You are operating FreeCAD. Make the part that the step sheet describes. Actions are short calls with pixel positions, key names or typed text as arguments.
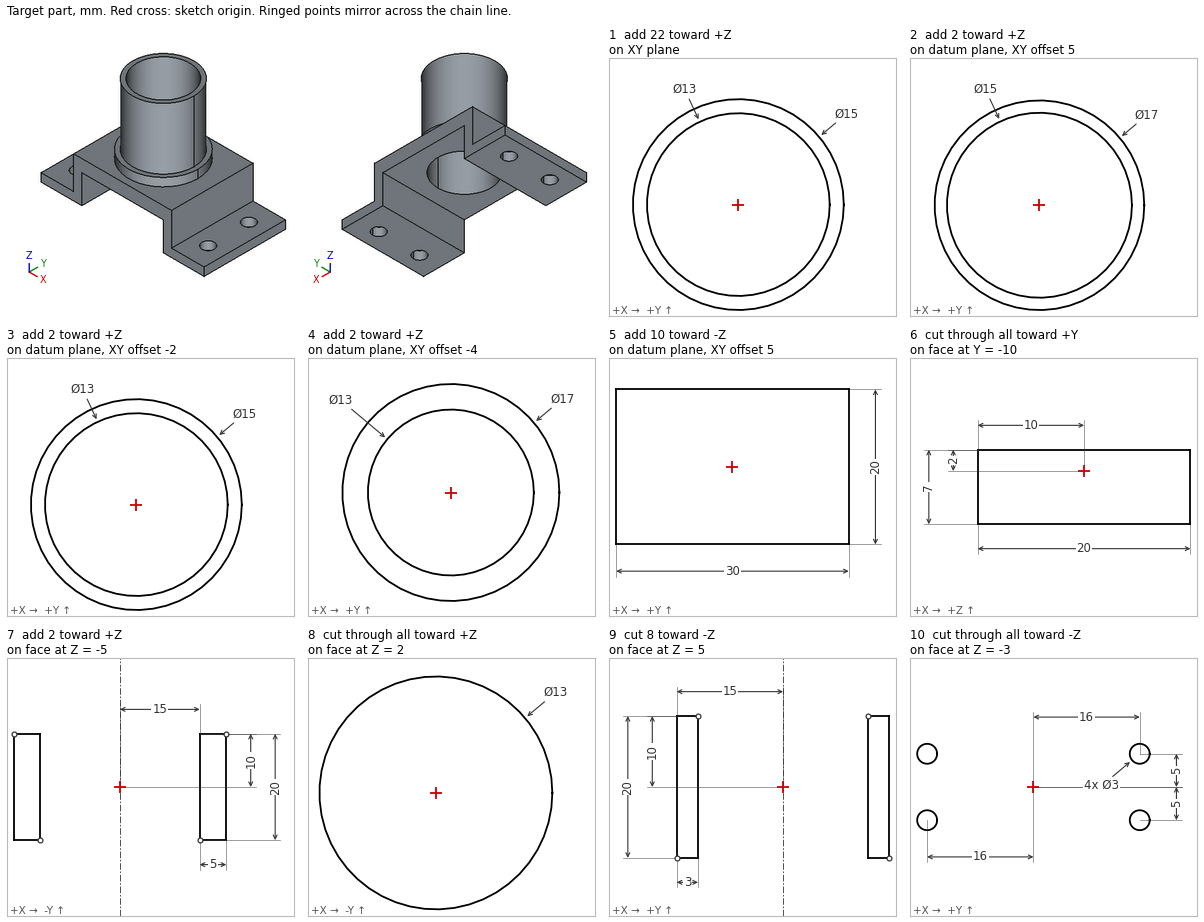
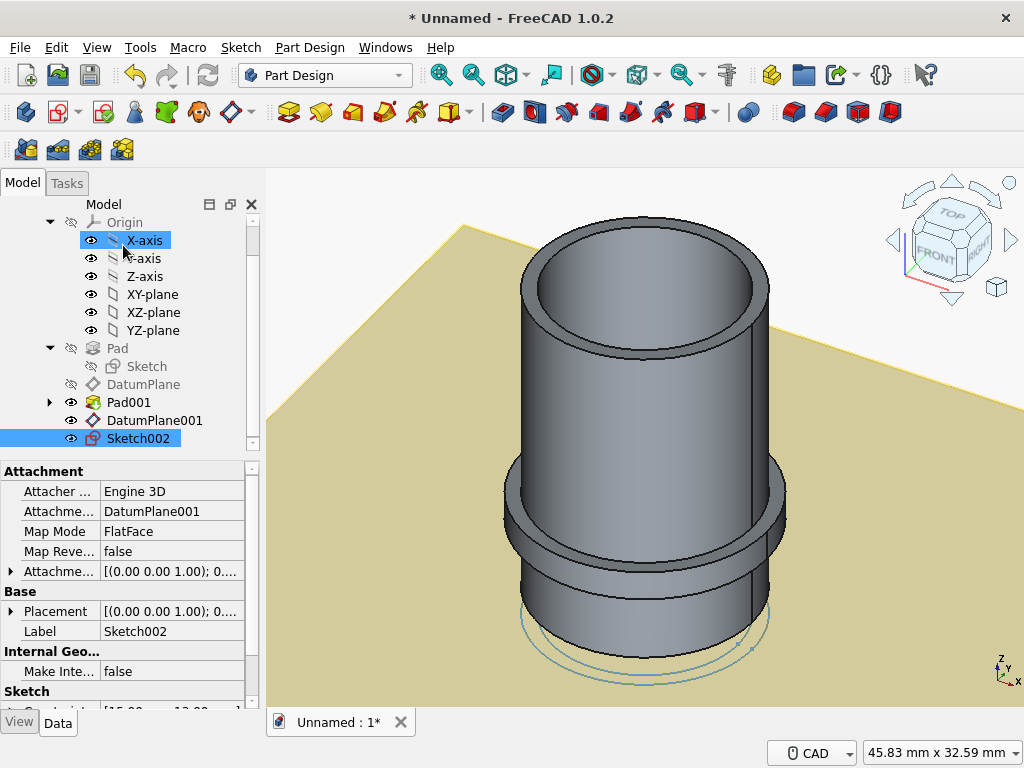
click(290, 112)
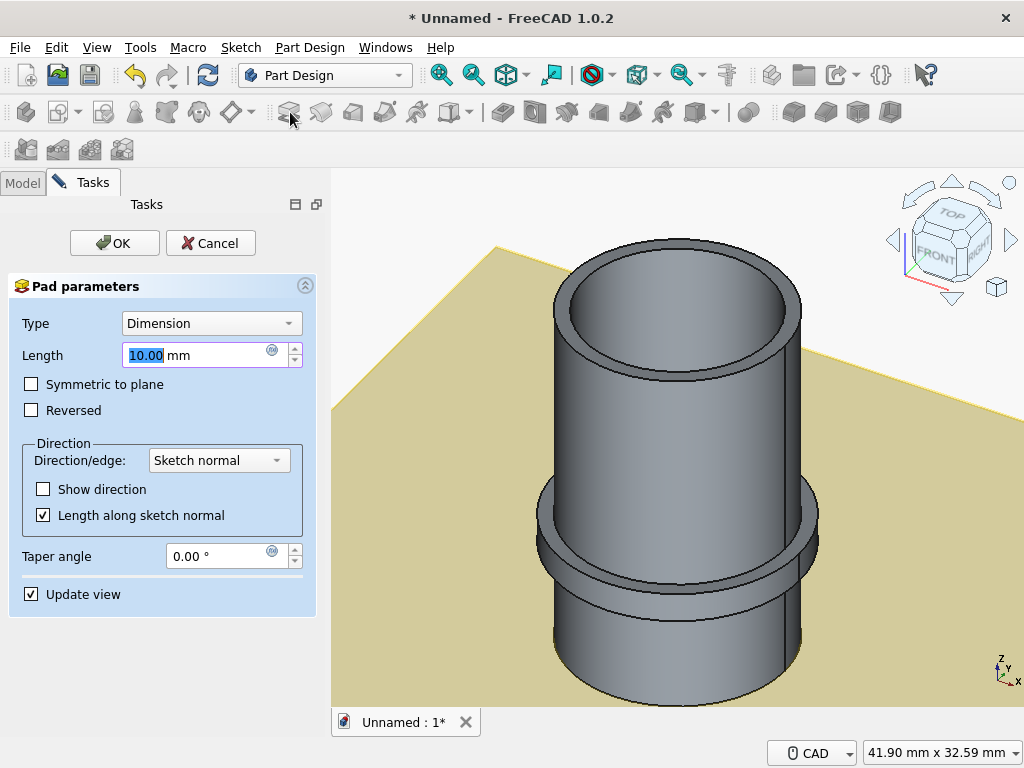
text(2)
key(Tab)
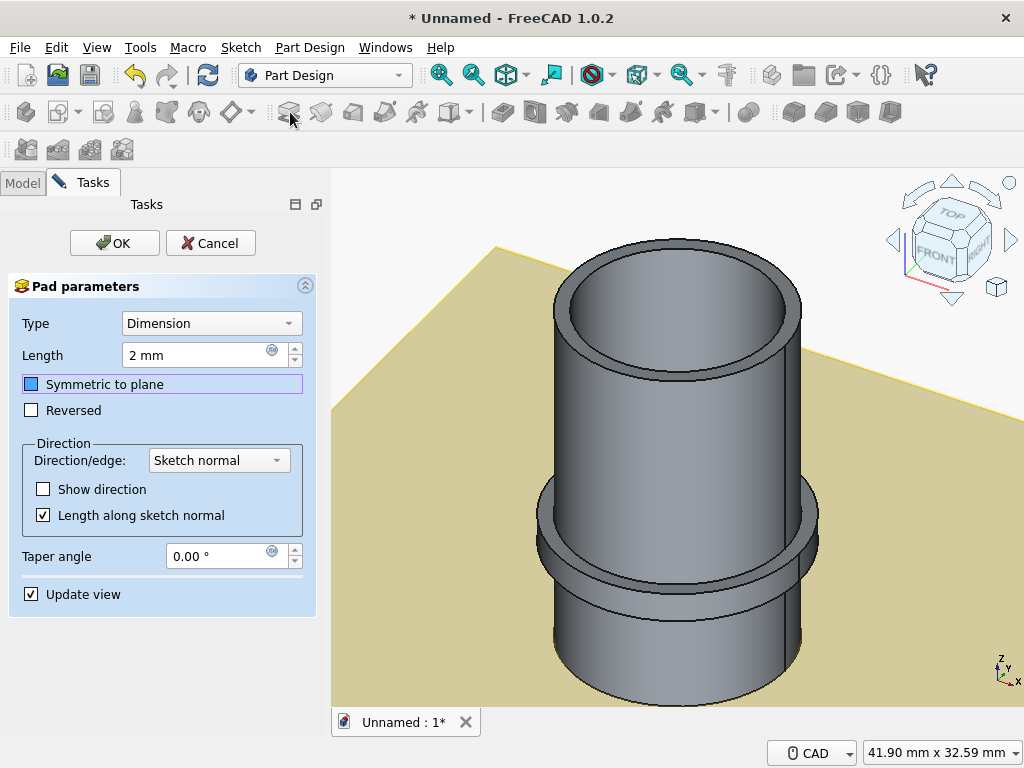
click(115, 243)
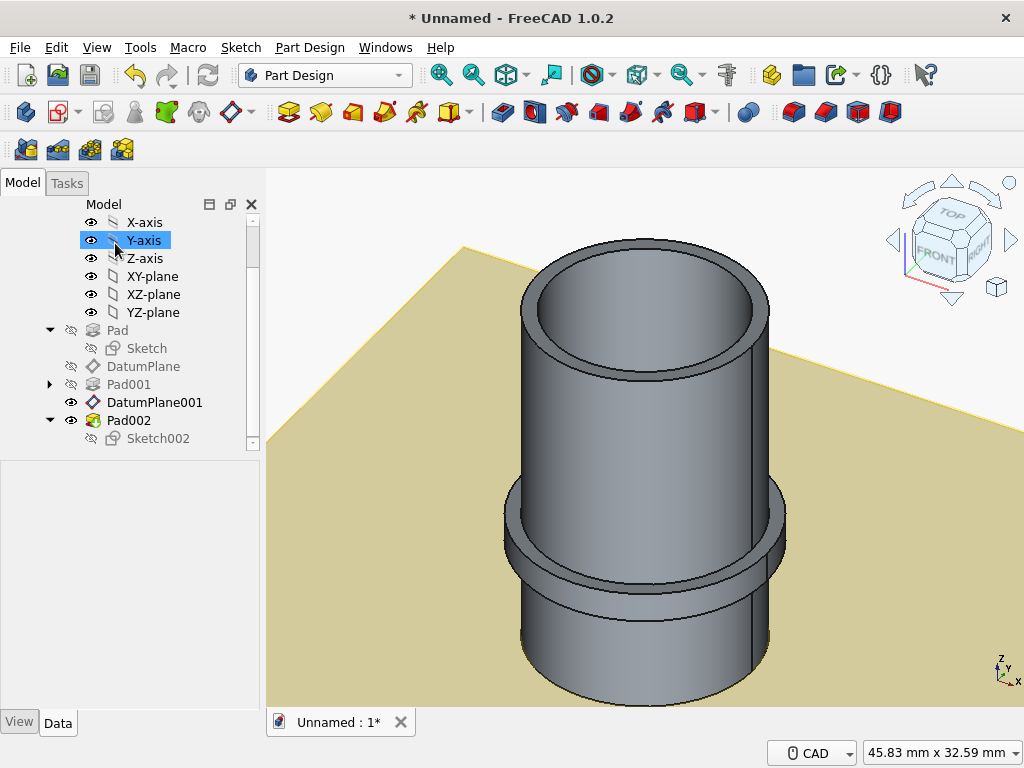
click(116, 402)
key(space)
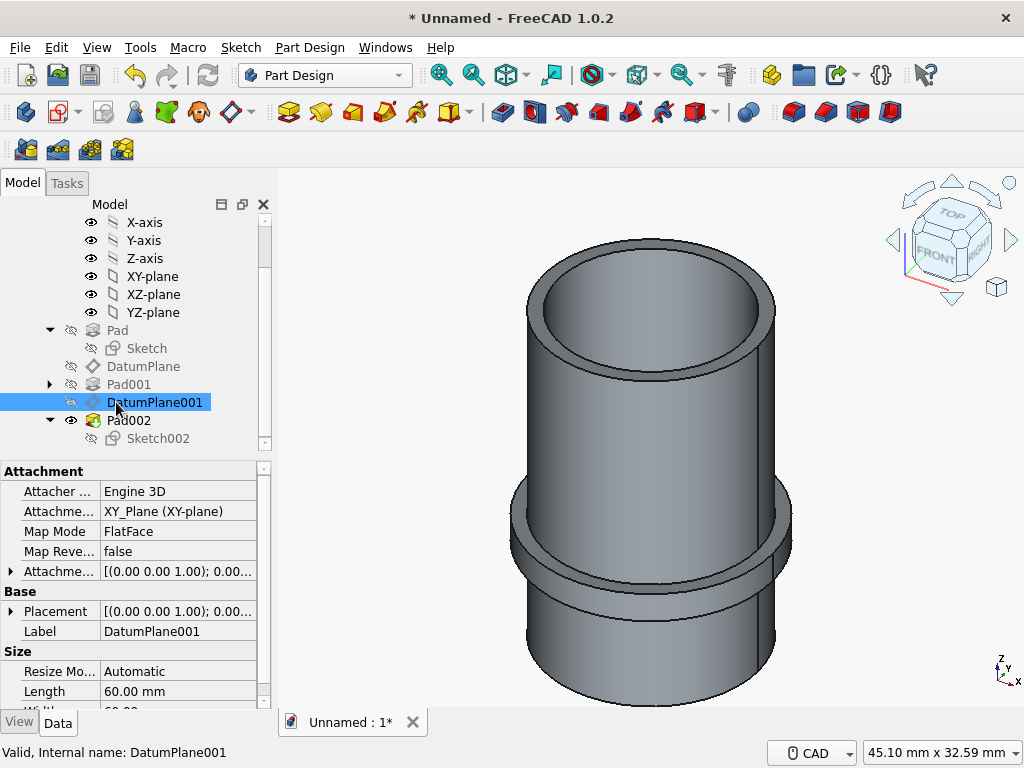
click(442, 76)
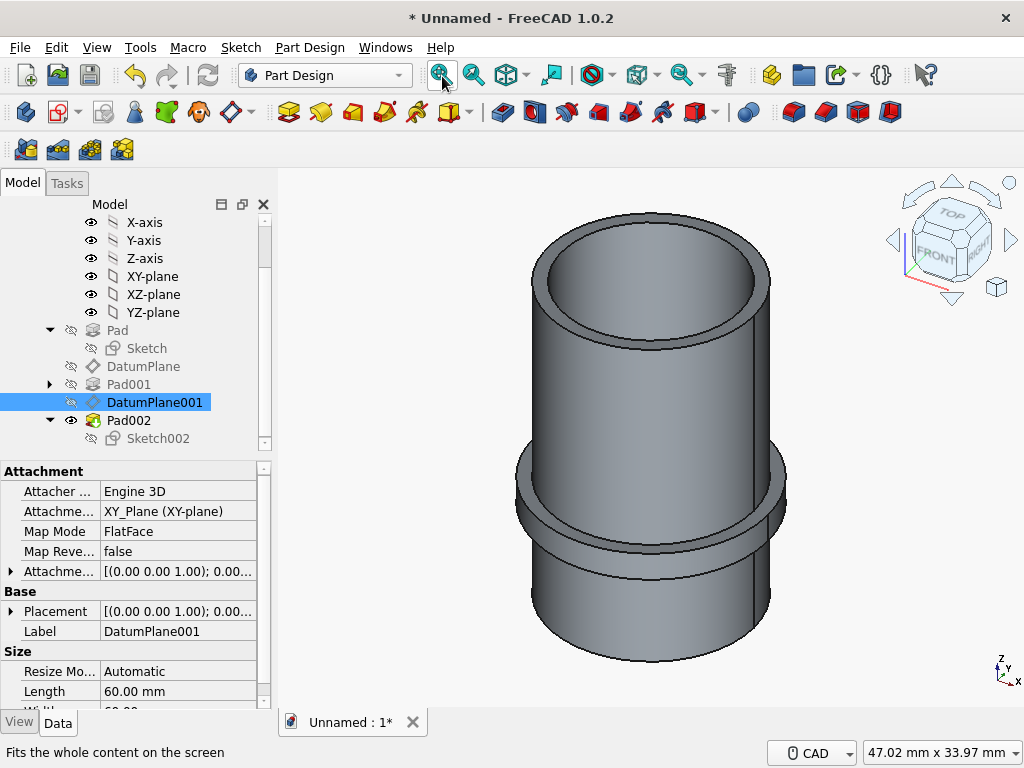
scroll(160, 326, down, 3)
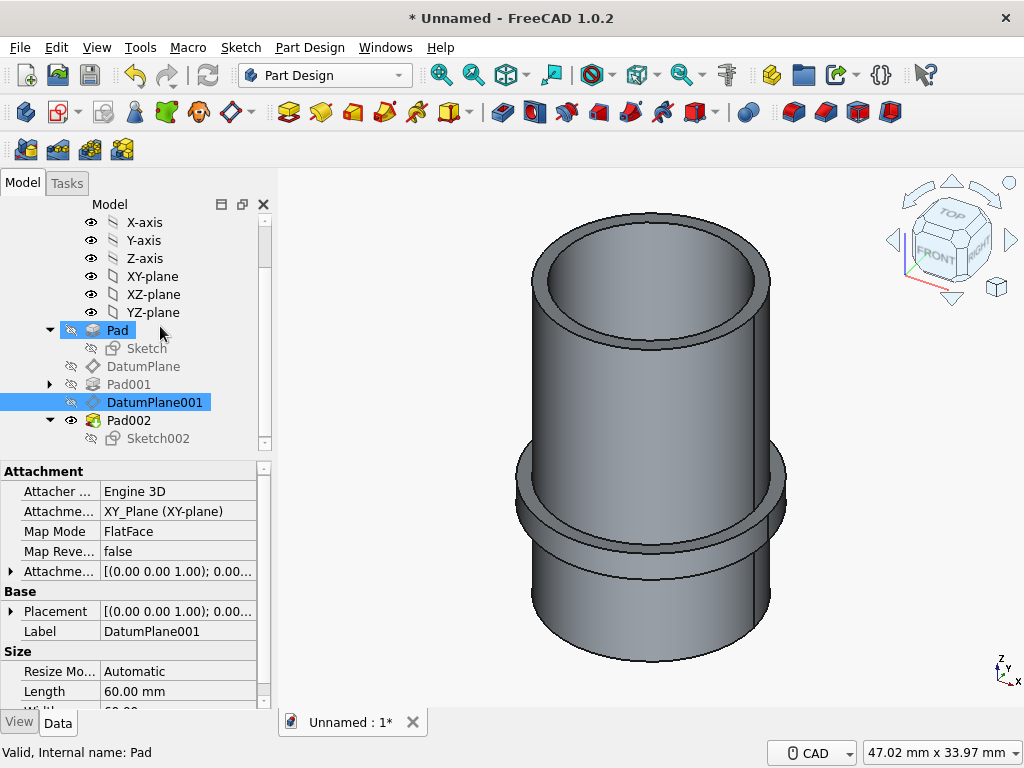
scroll(160, 326, up, 15)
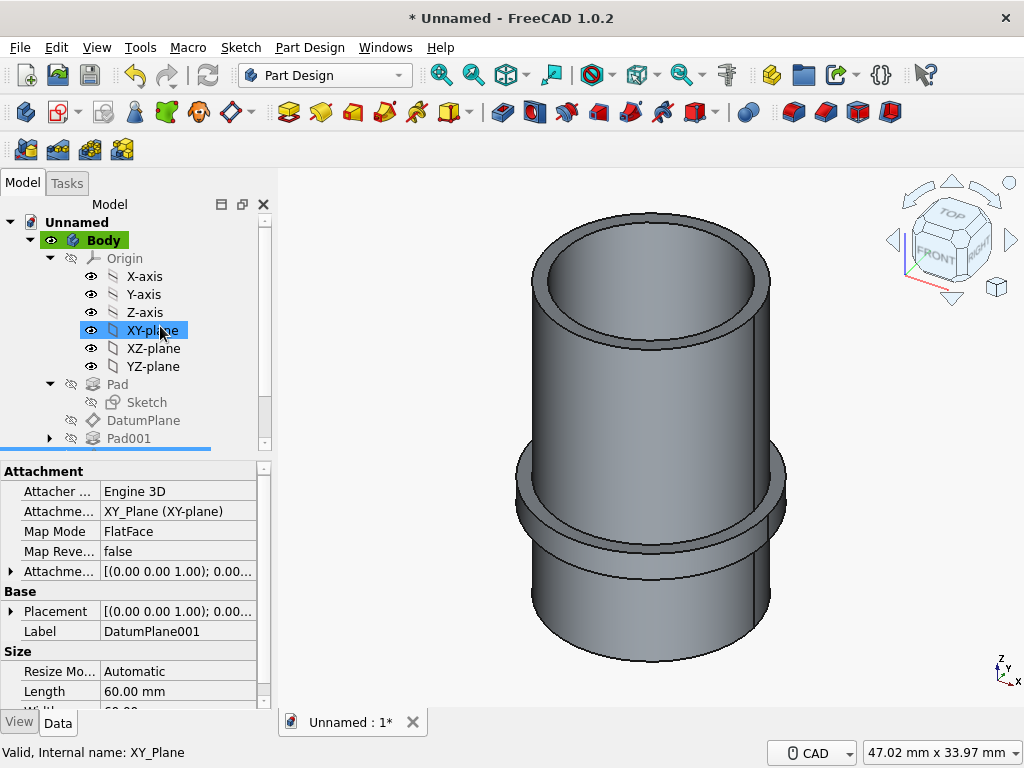
click(136, 330)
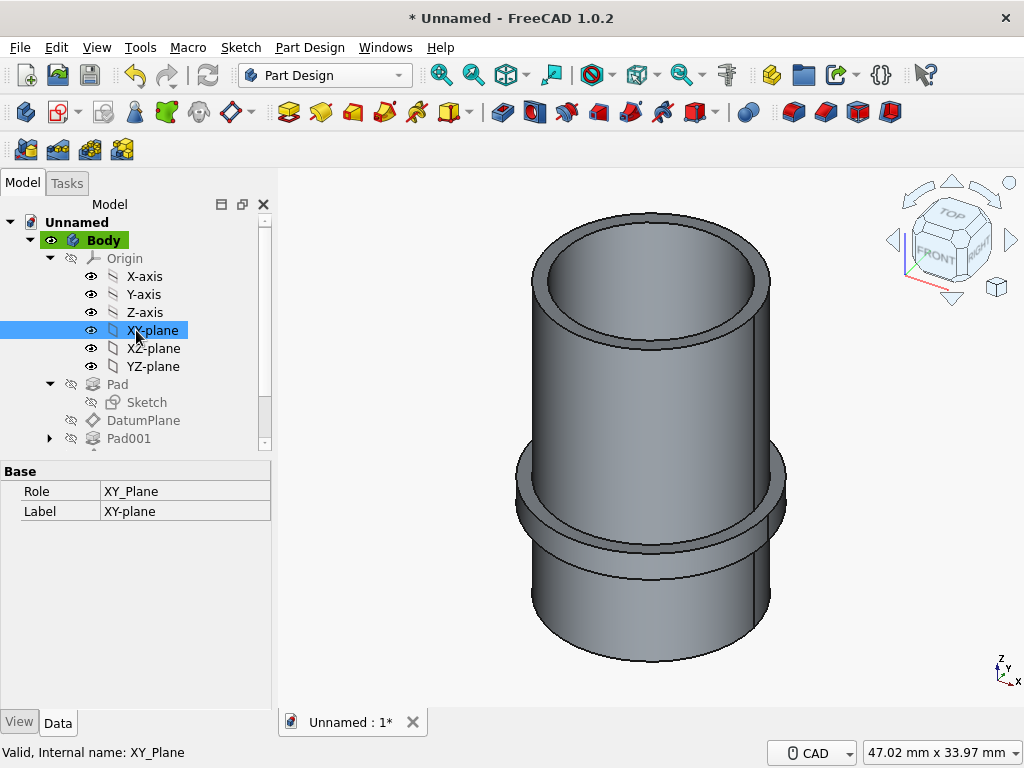
click(232, 112)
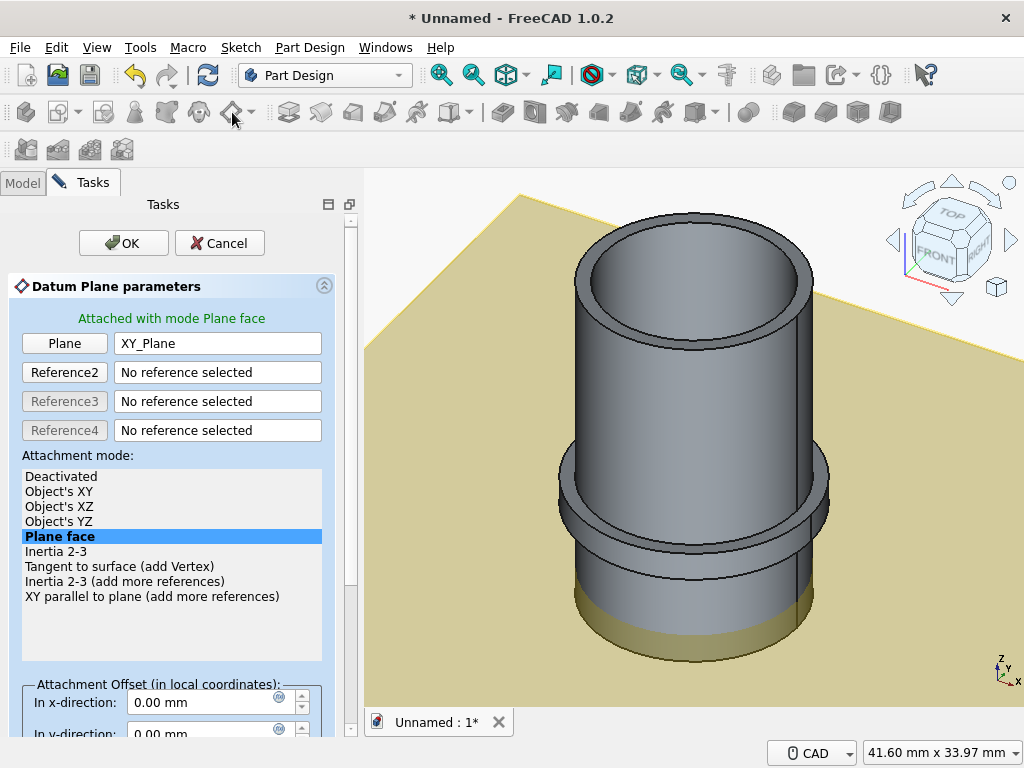
scroll(351, 475, down, 2)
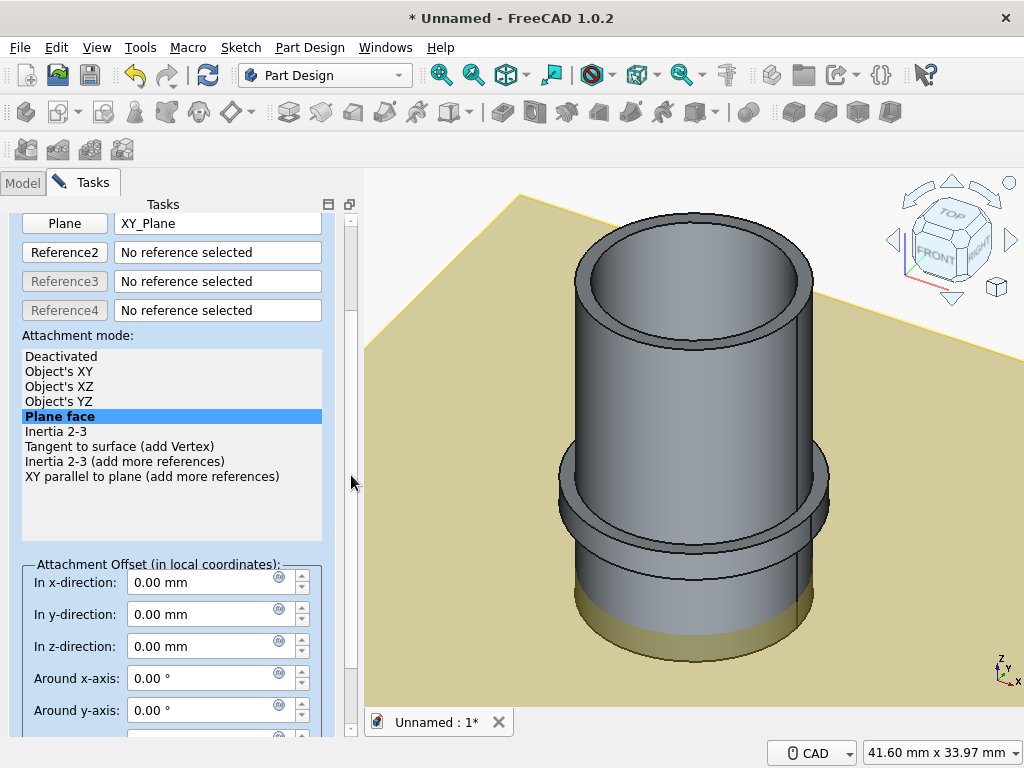
triple_click(210, 646)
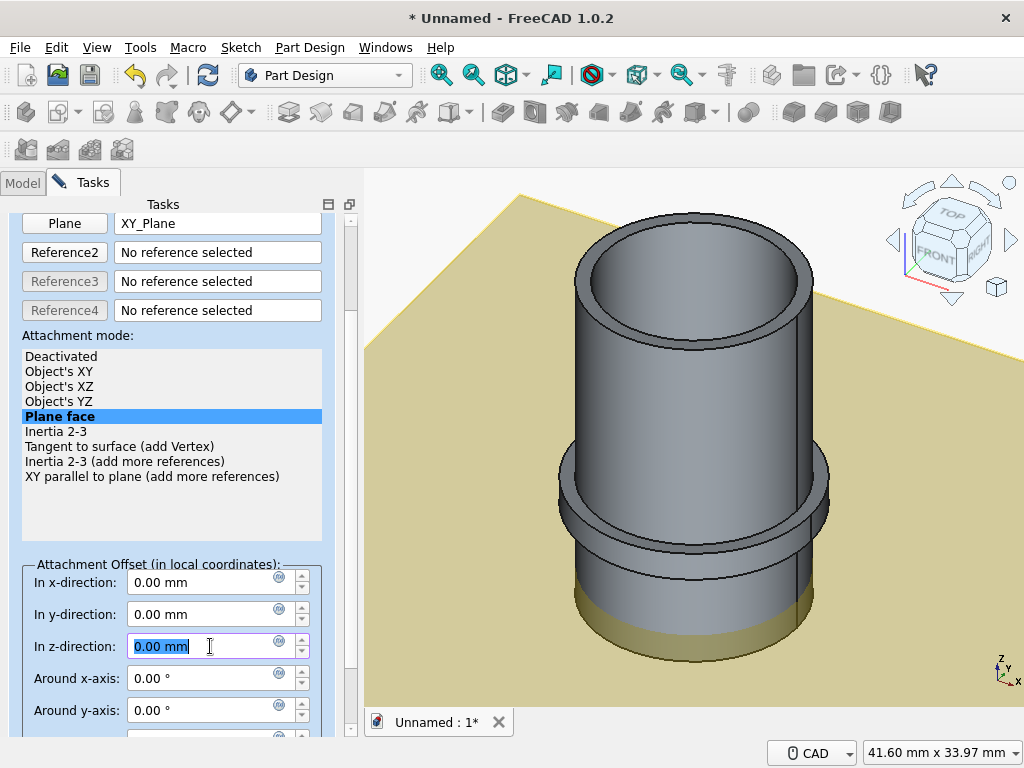
text(-4)
key(Tab)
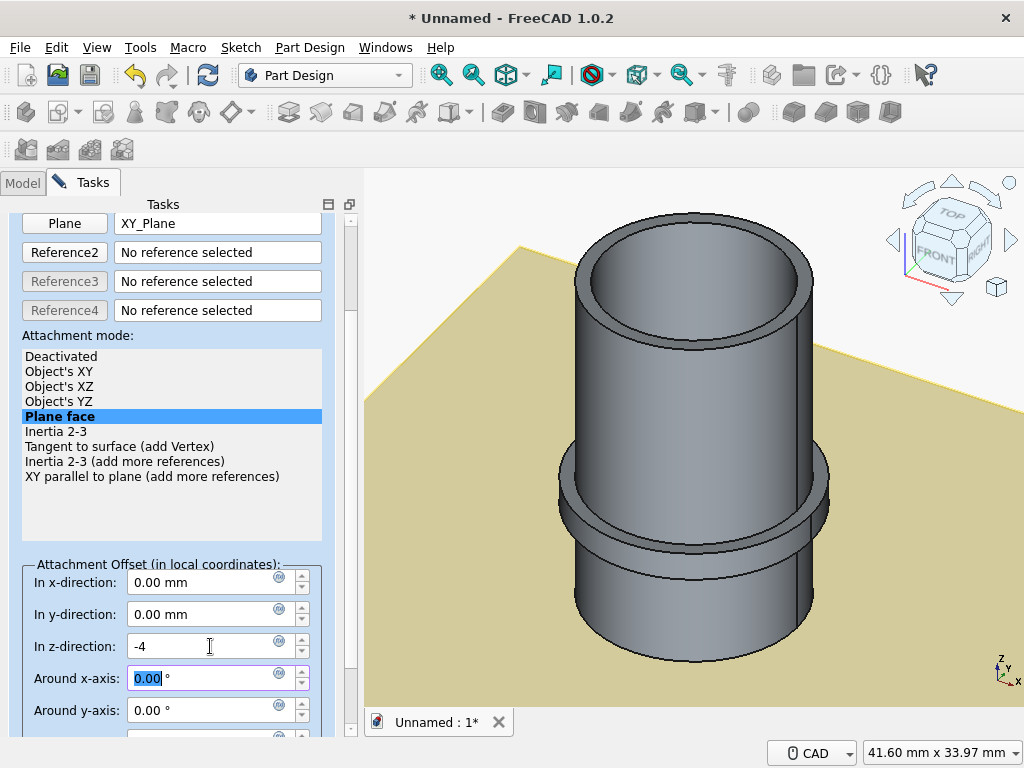
scroll(351, 475, up, 3)